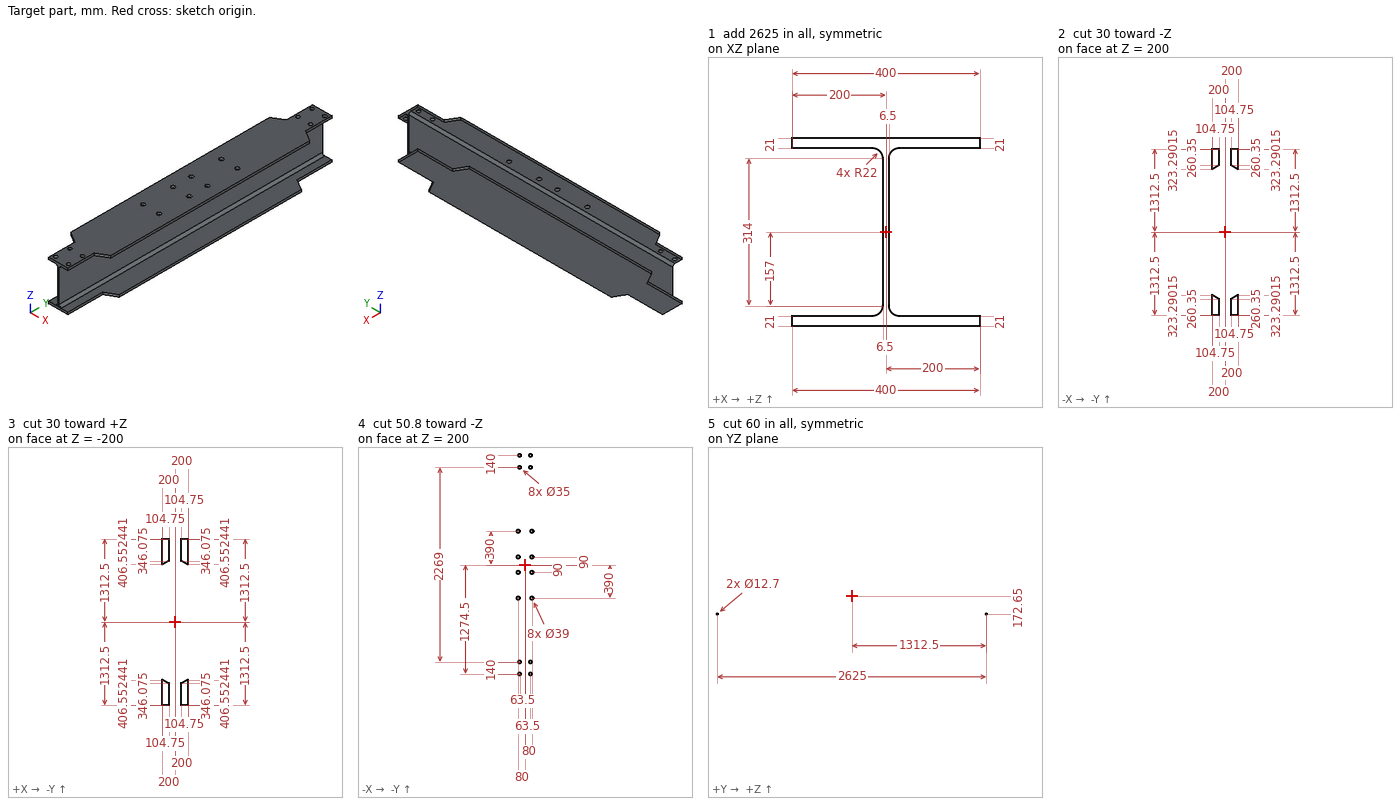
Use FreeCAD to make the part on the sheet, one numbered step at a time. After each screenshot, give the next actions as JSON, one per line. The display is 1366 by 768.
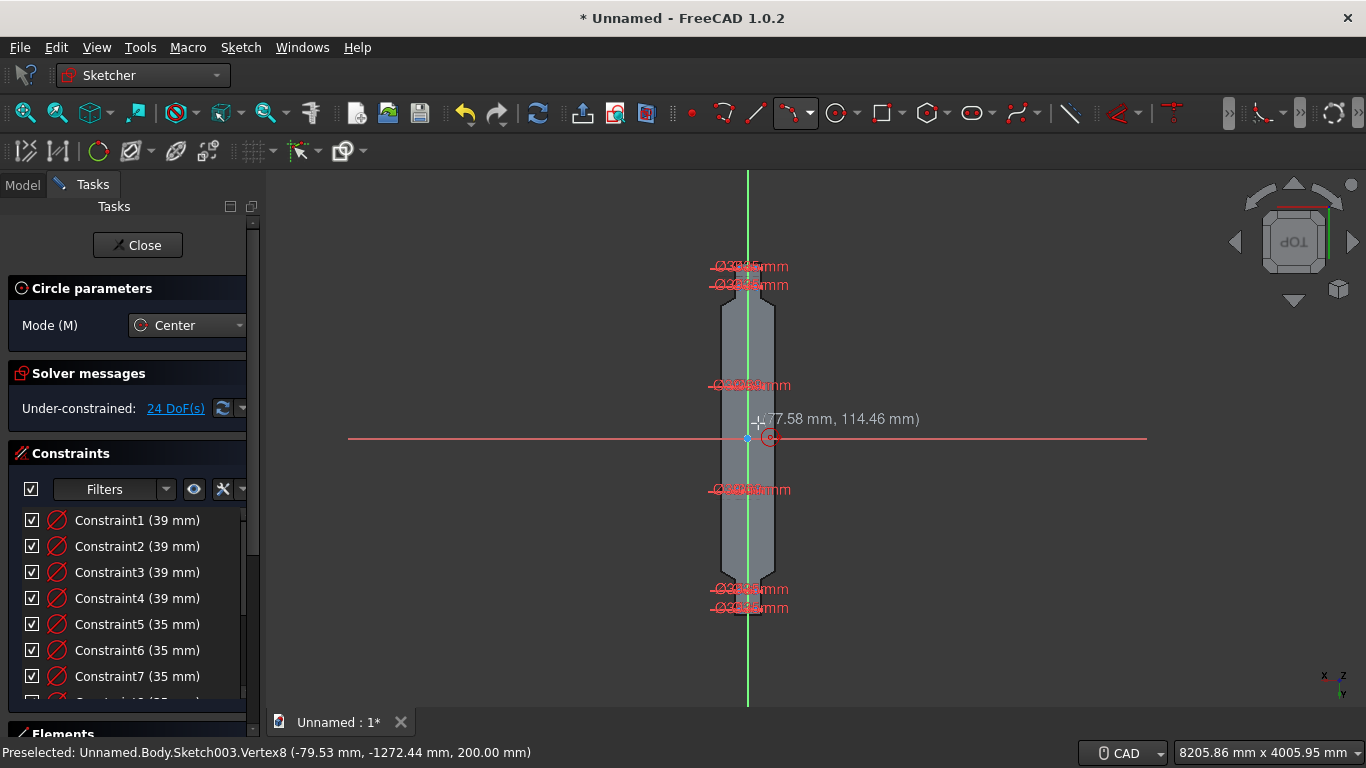
{"action": "scroll", "coordinate": [759, 451], "scroll_direction": "up", "scroll_amount": 2}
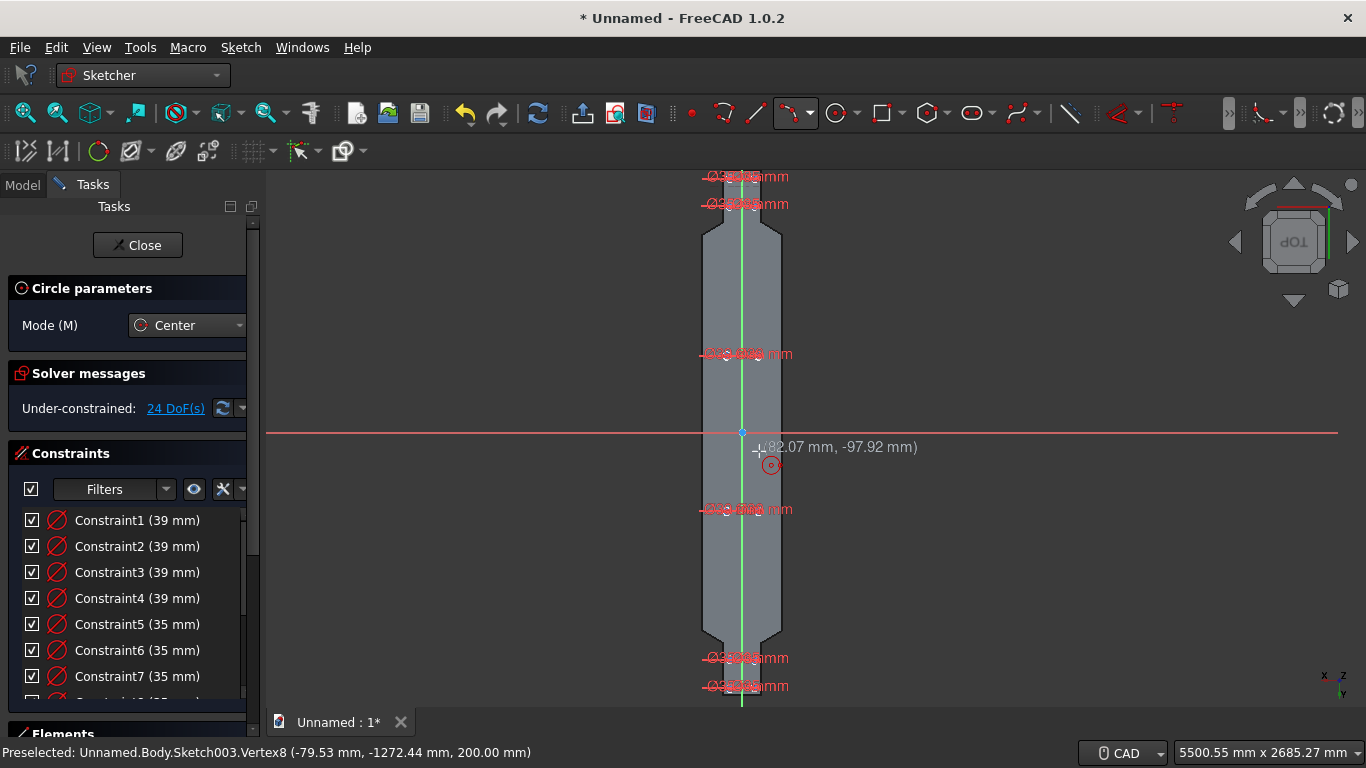
{"action": "left_click", "coordinate": [758, 451]}
{"action": "mouse_move", "coordinate": [761, 448]}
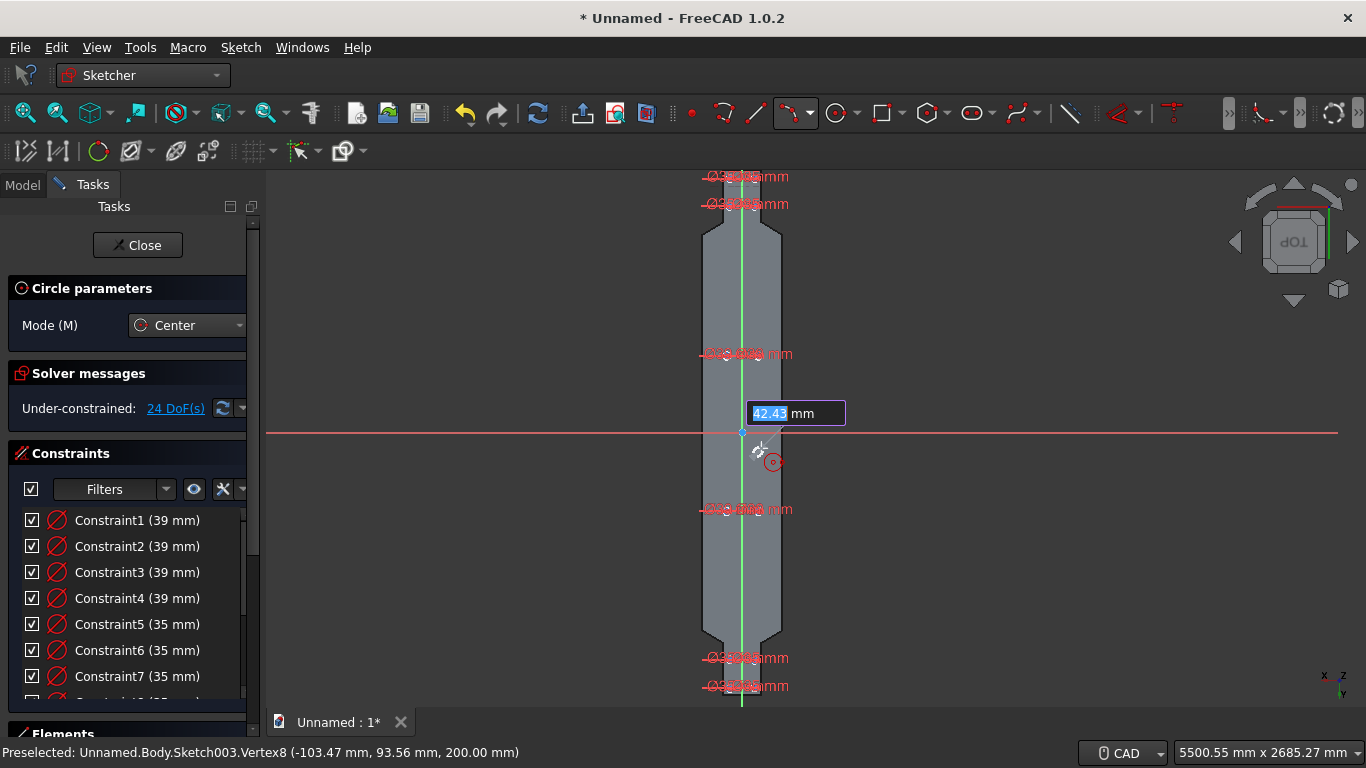
{"action": "type", "text": "39"}
{"action": "key", "text": "Return"}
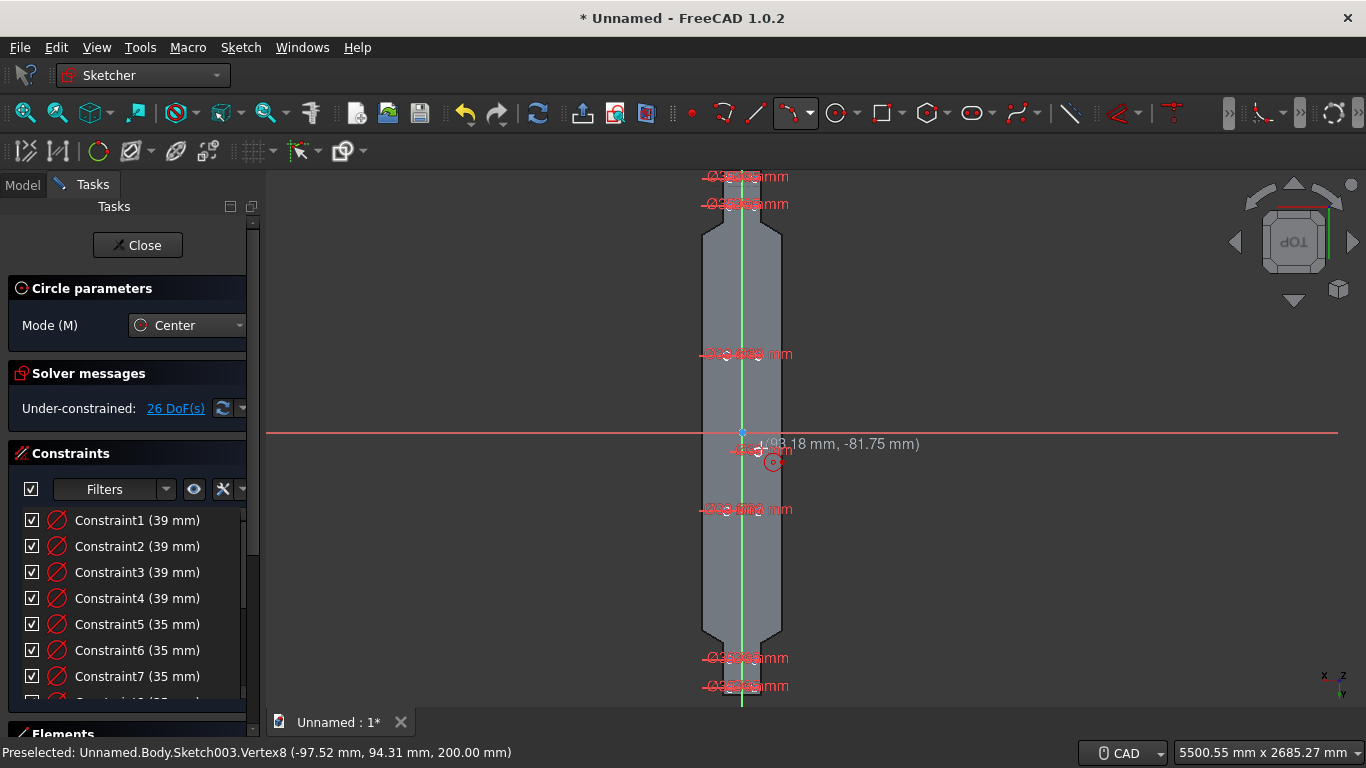
{"action": "scroll", "coordinate": [726, 451], "scroll_direction": "up", "scroll_amount": 9}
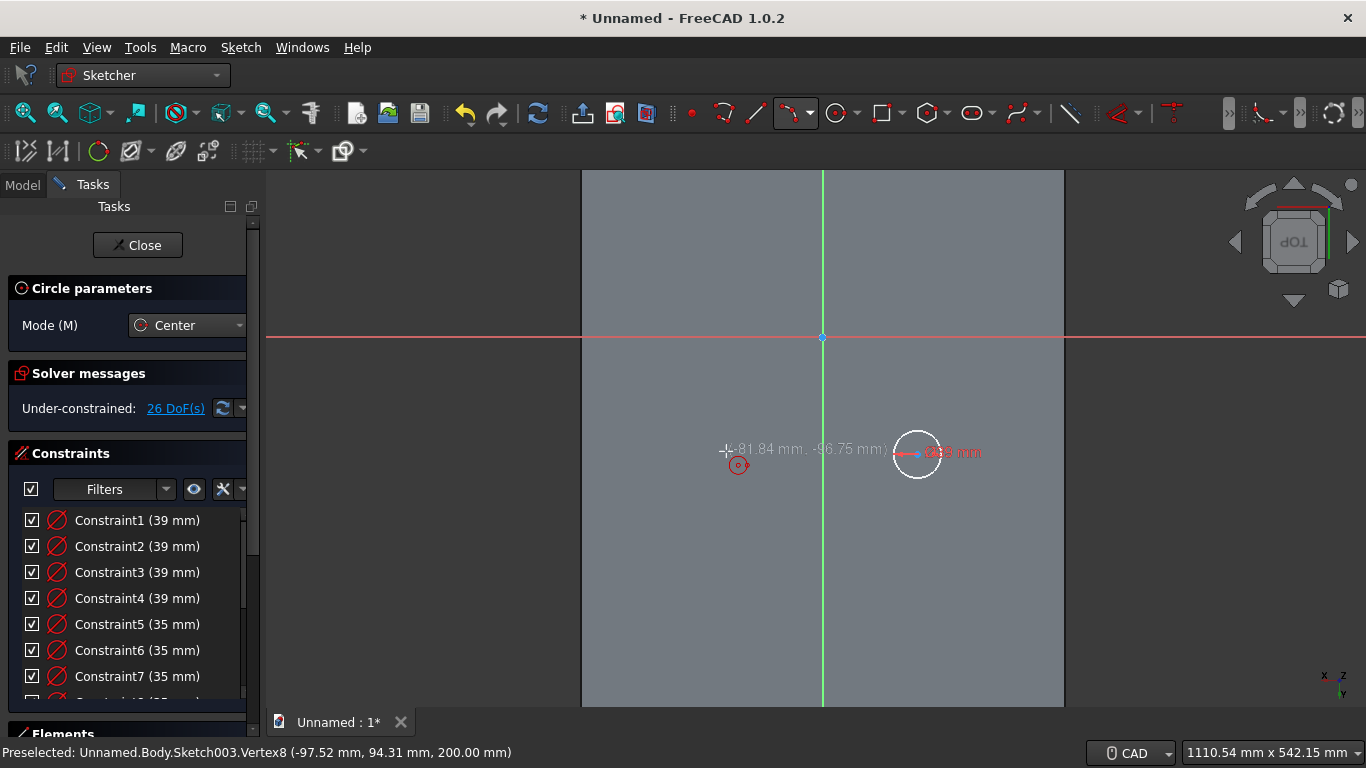
{"action": "scroll", "coordinate": [738, 451], "scroll_direction": "down", "scroll_amount": 11}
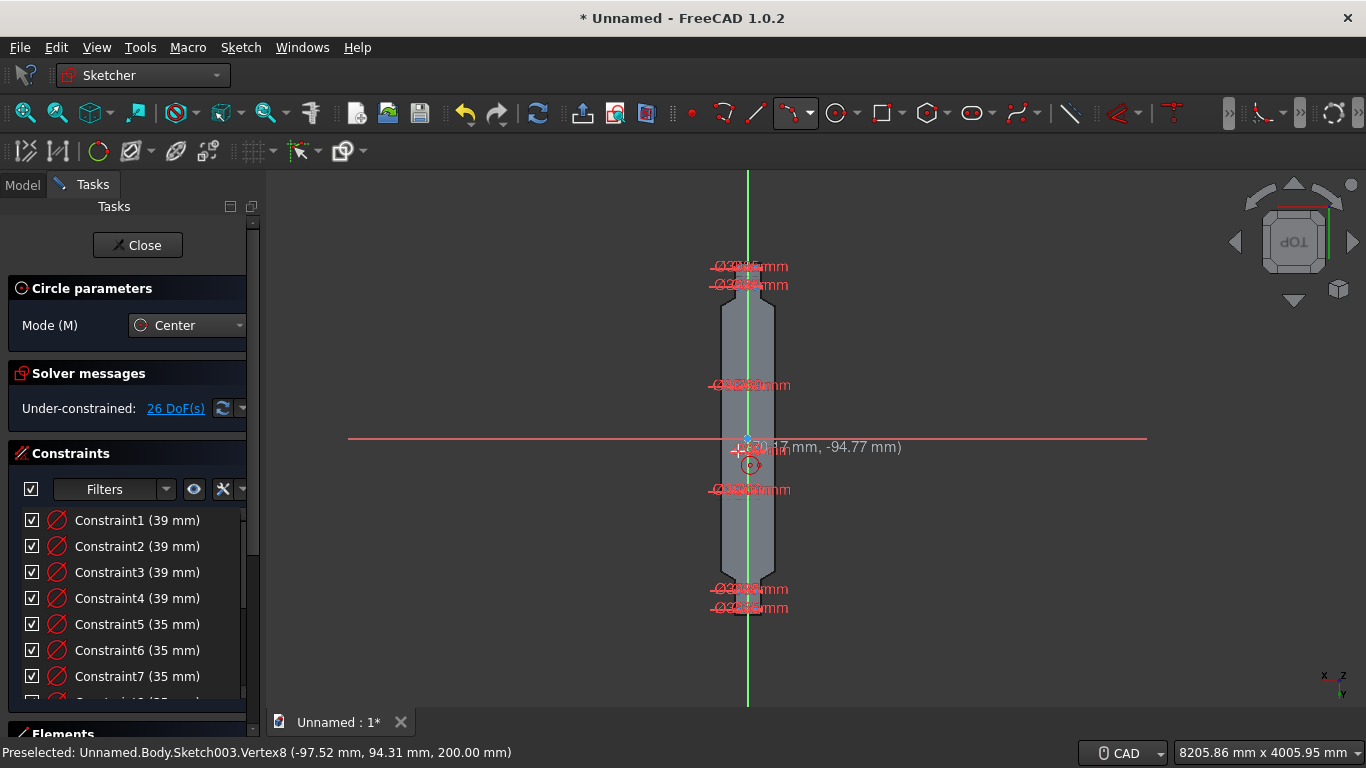
{"action": "scroll", "coordinate": [737, 451], "scroll_direction": "up", "scroll_amount": 2}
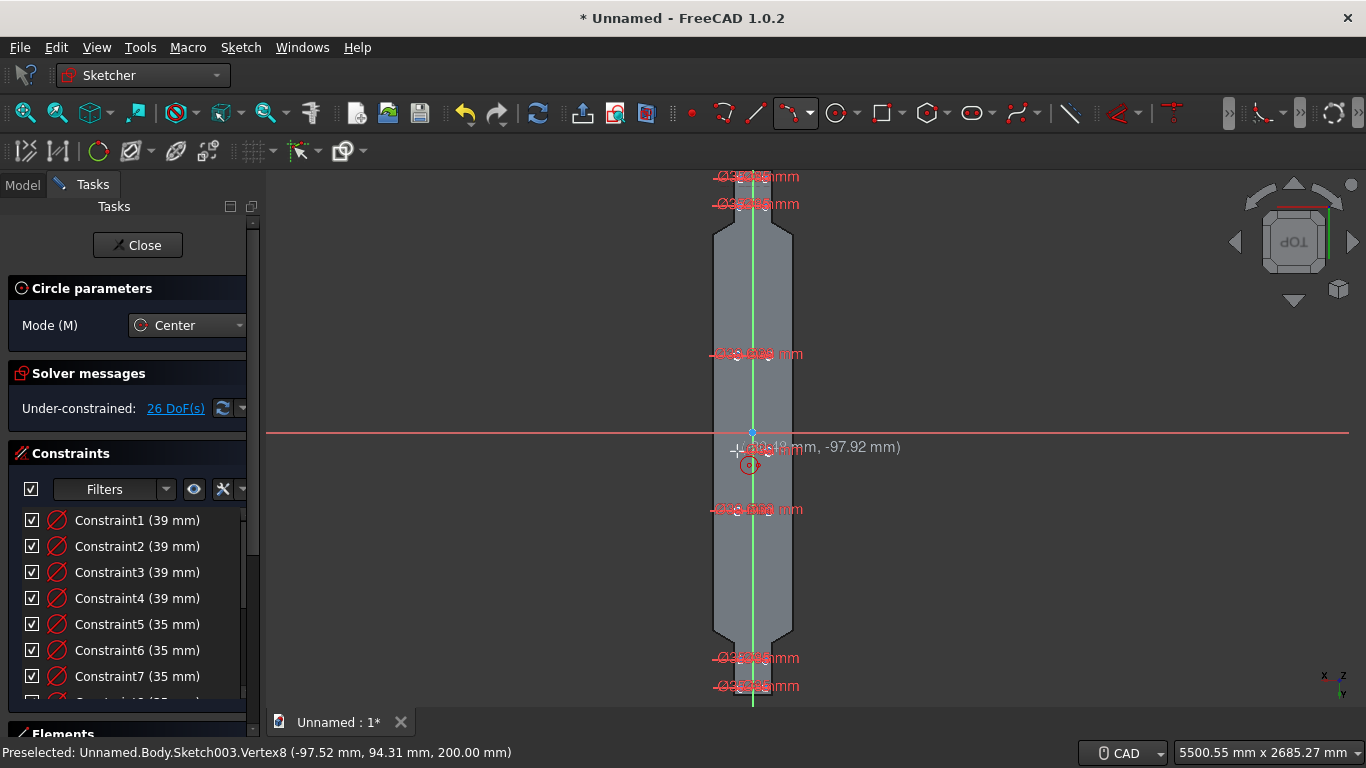
{"action": "left_click", "coordinate": [737, 451]}
{"action": "mouse_move", "coordinate": [734, 448]}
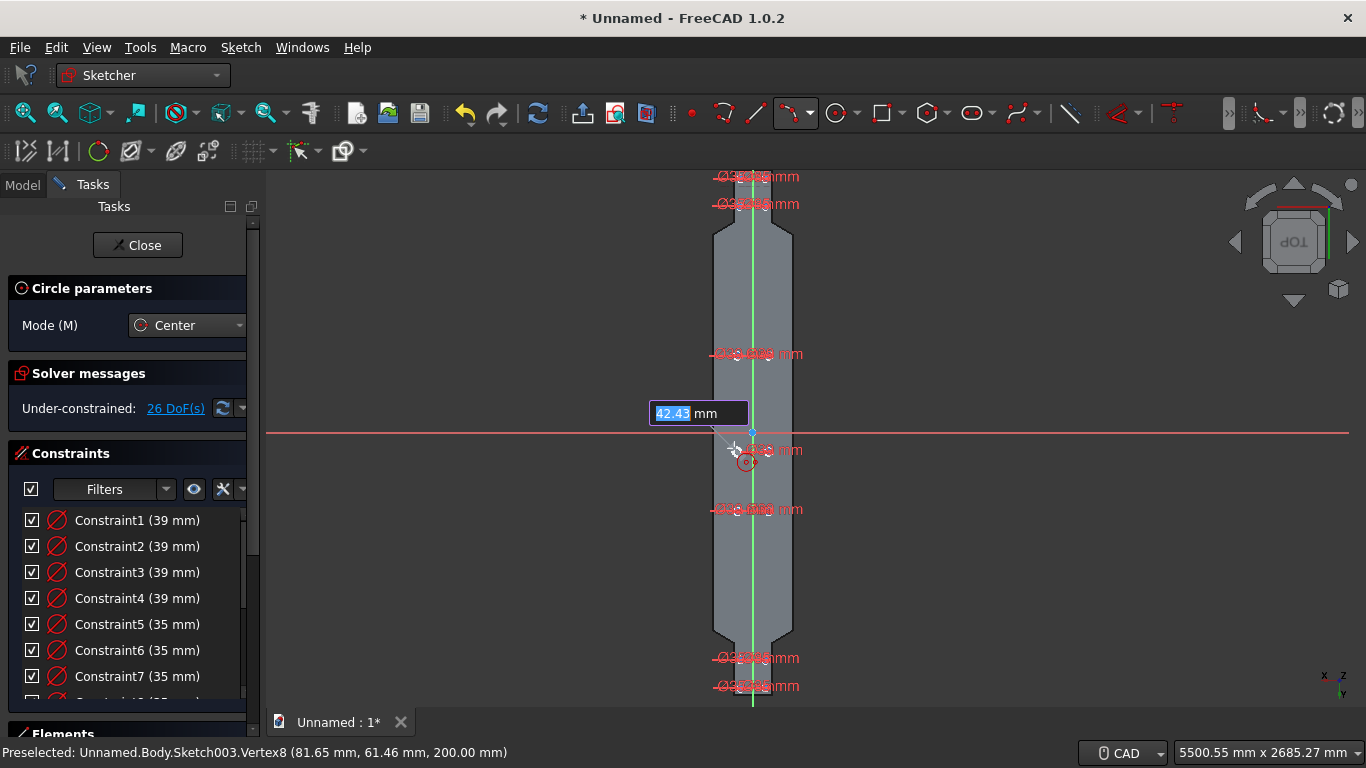
{"action": "type", "text": "39"}
{"action": "key", "text": "Return"}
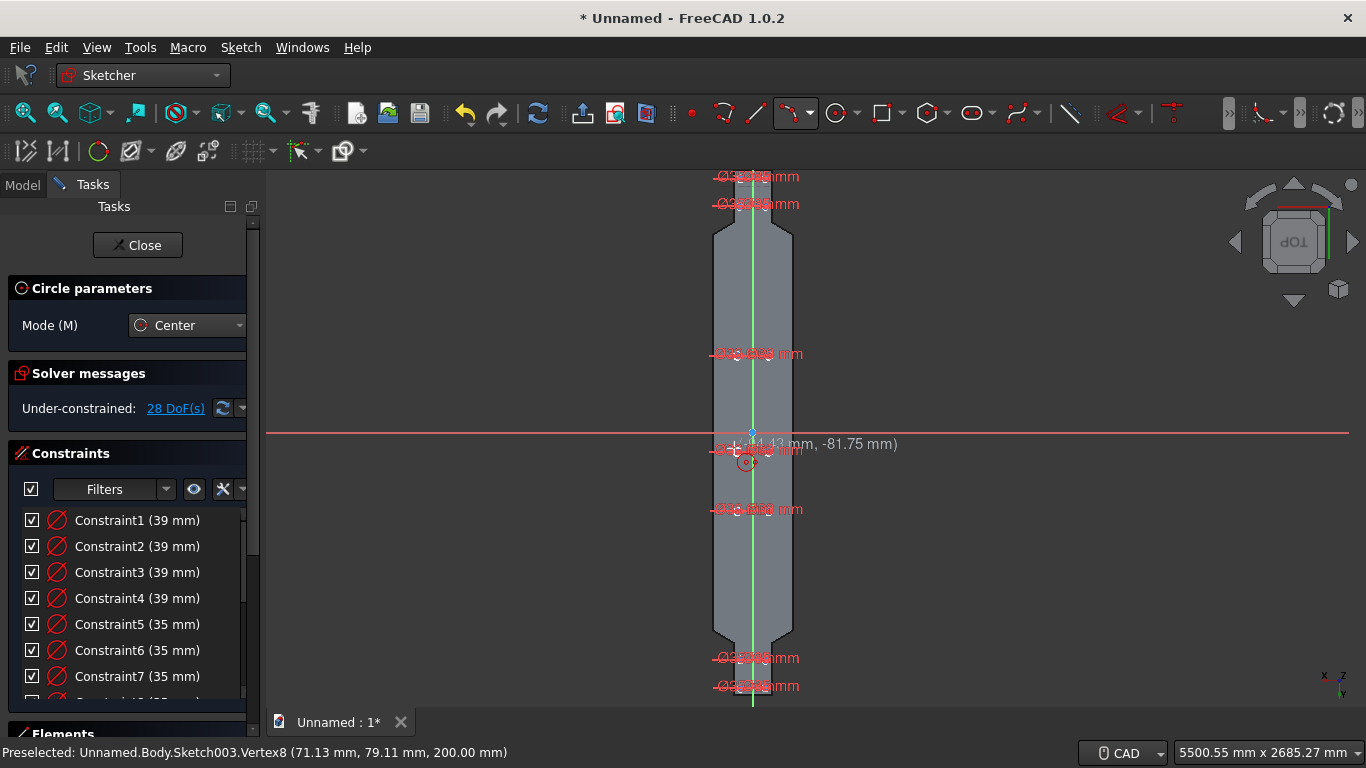
{"action": "scroll", "coordinate": [769, 415], "scroll_direction": "up", "scroll_amount": 9}